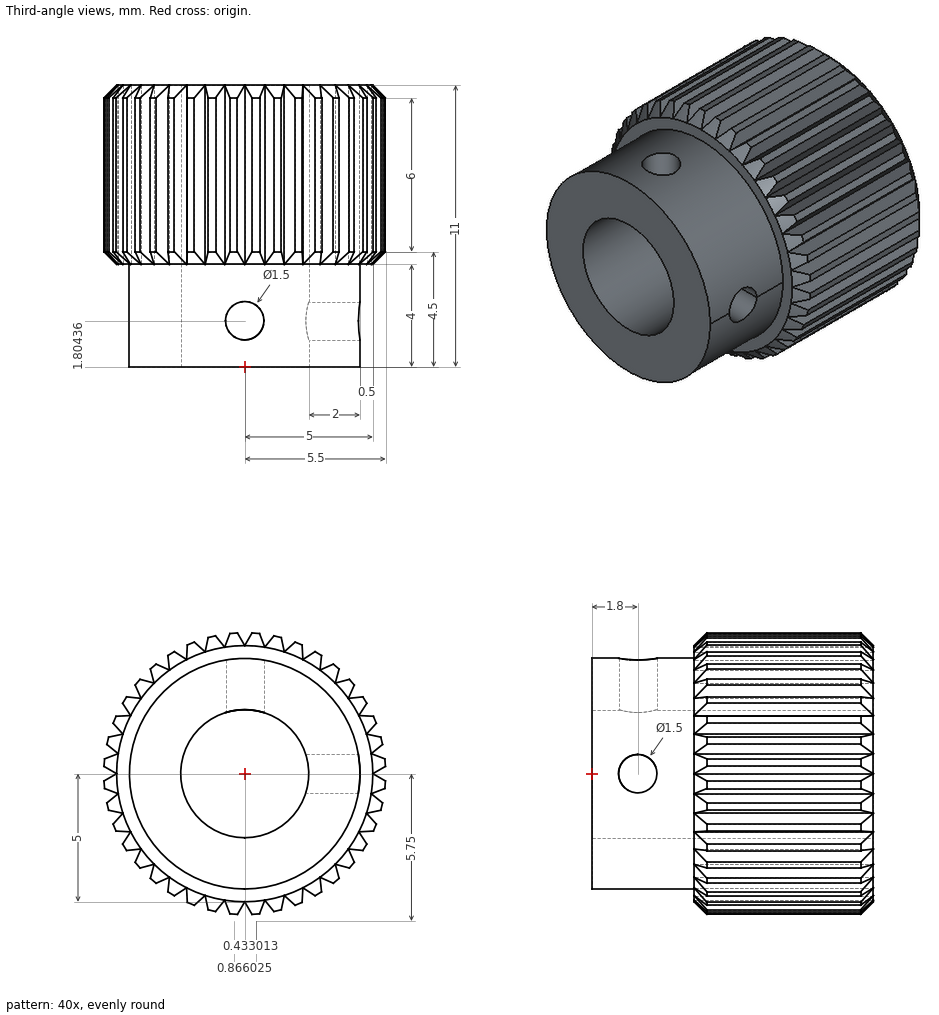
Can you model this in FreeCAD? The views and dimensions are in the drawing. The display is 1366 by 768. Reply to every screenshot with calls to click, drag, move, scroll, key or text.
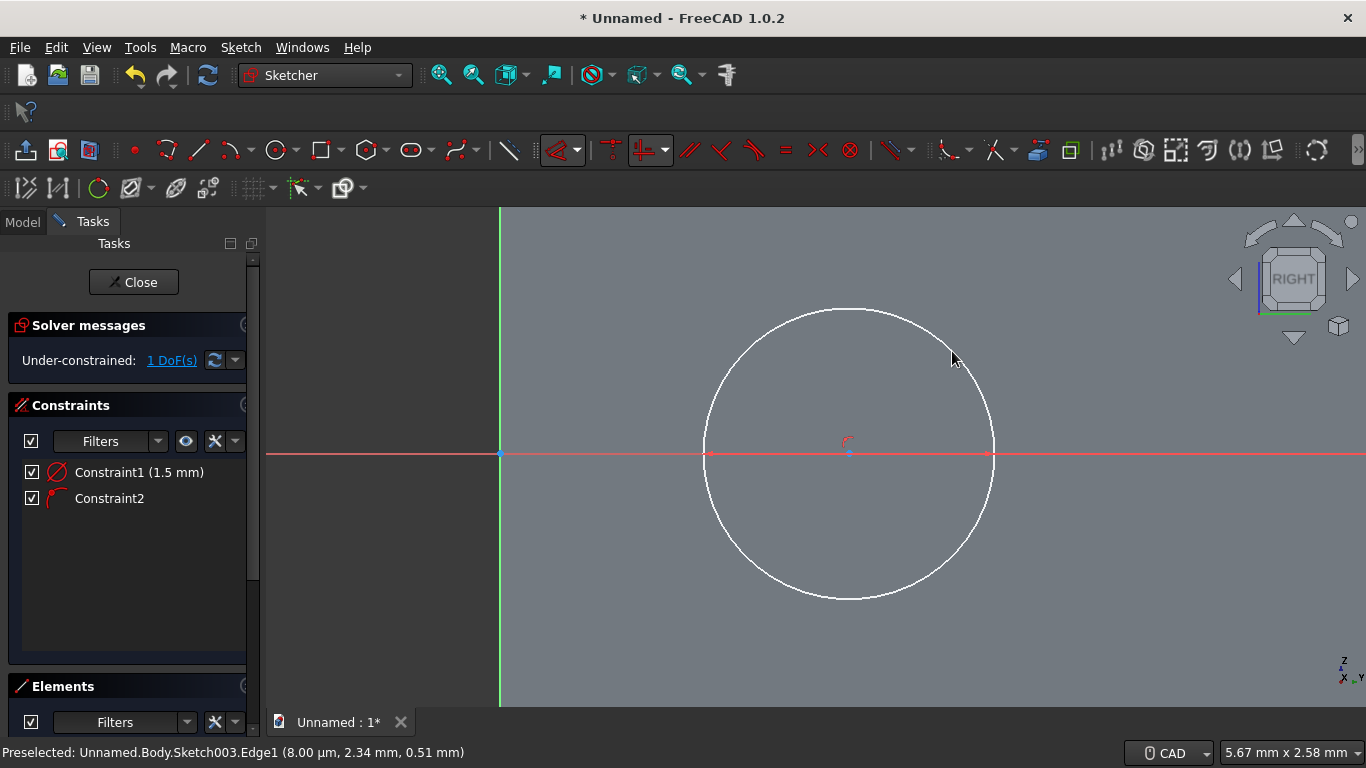
click(849, 454)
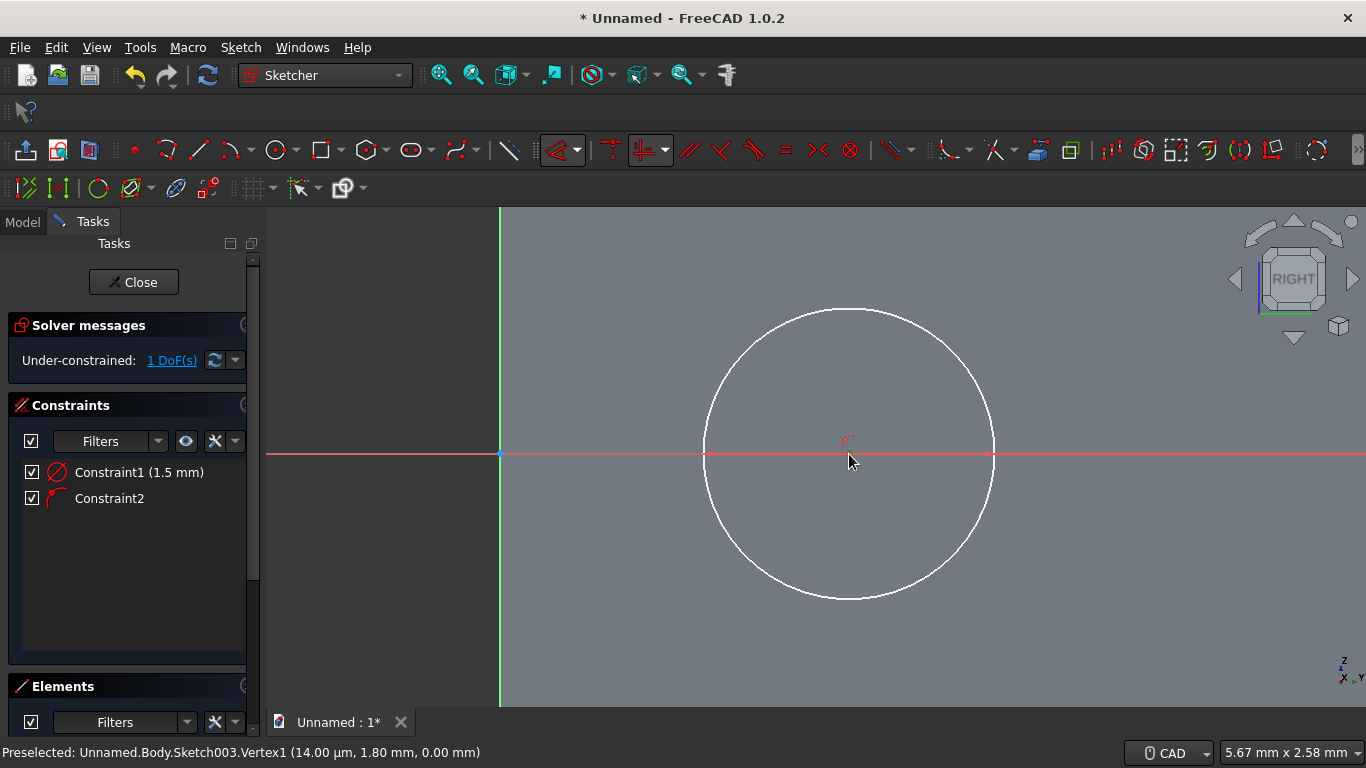
key(l)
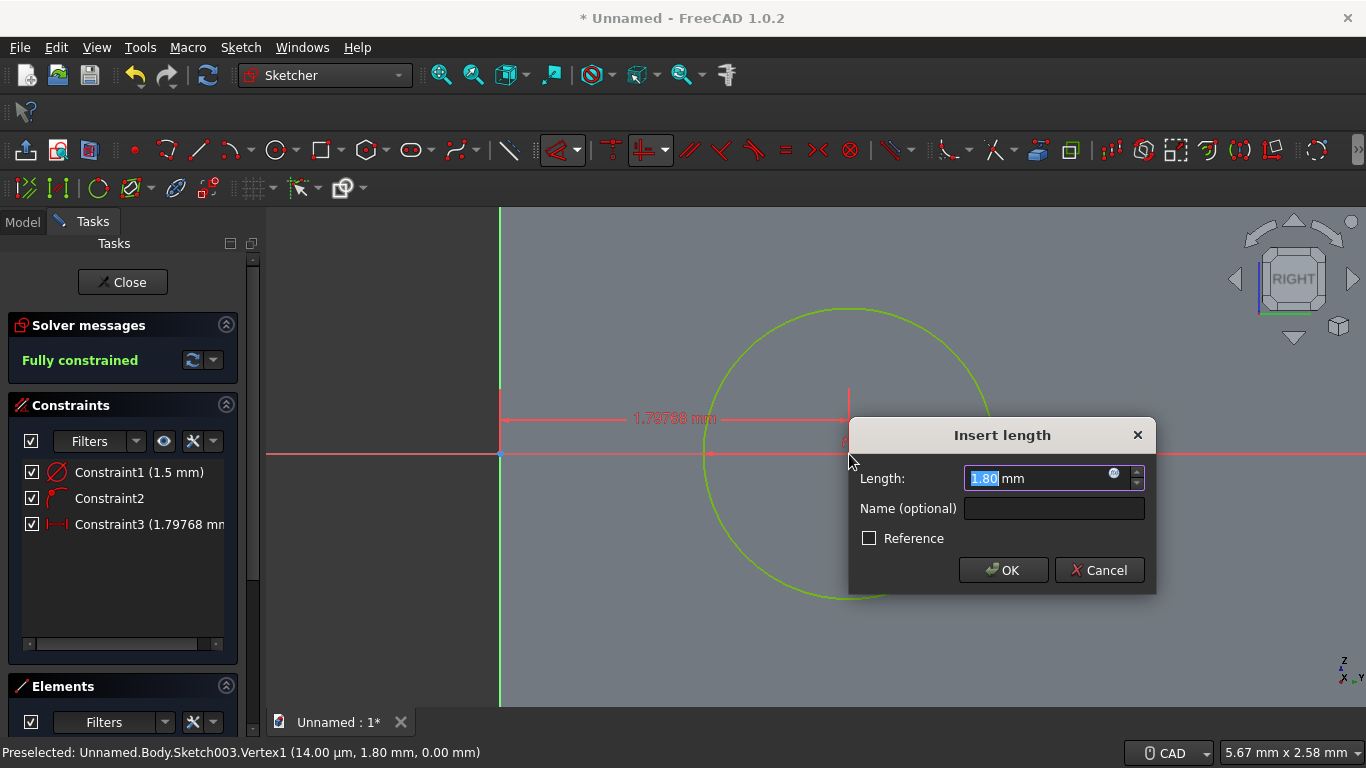
text(1.8)
key(Return)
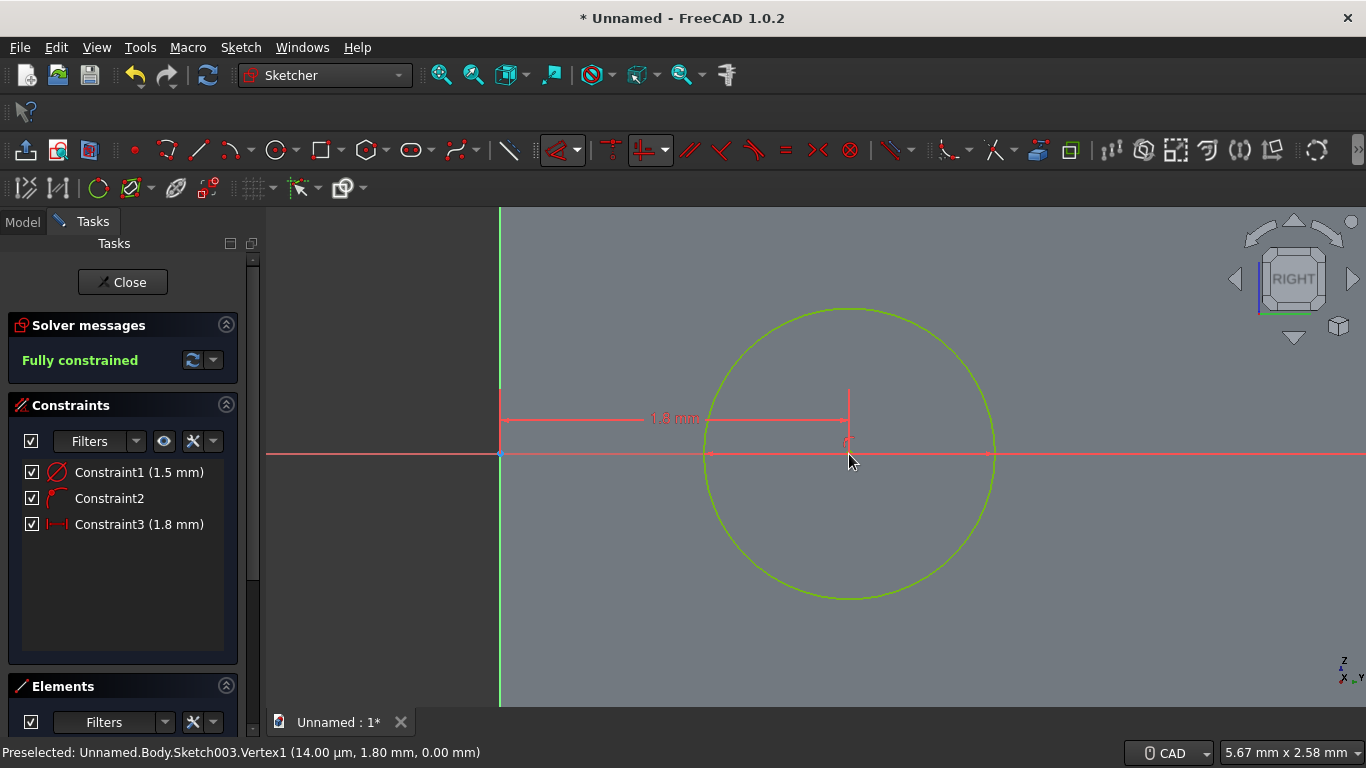
click(123, 282)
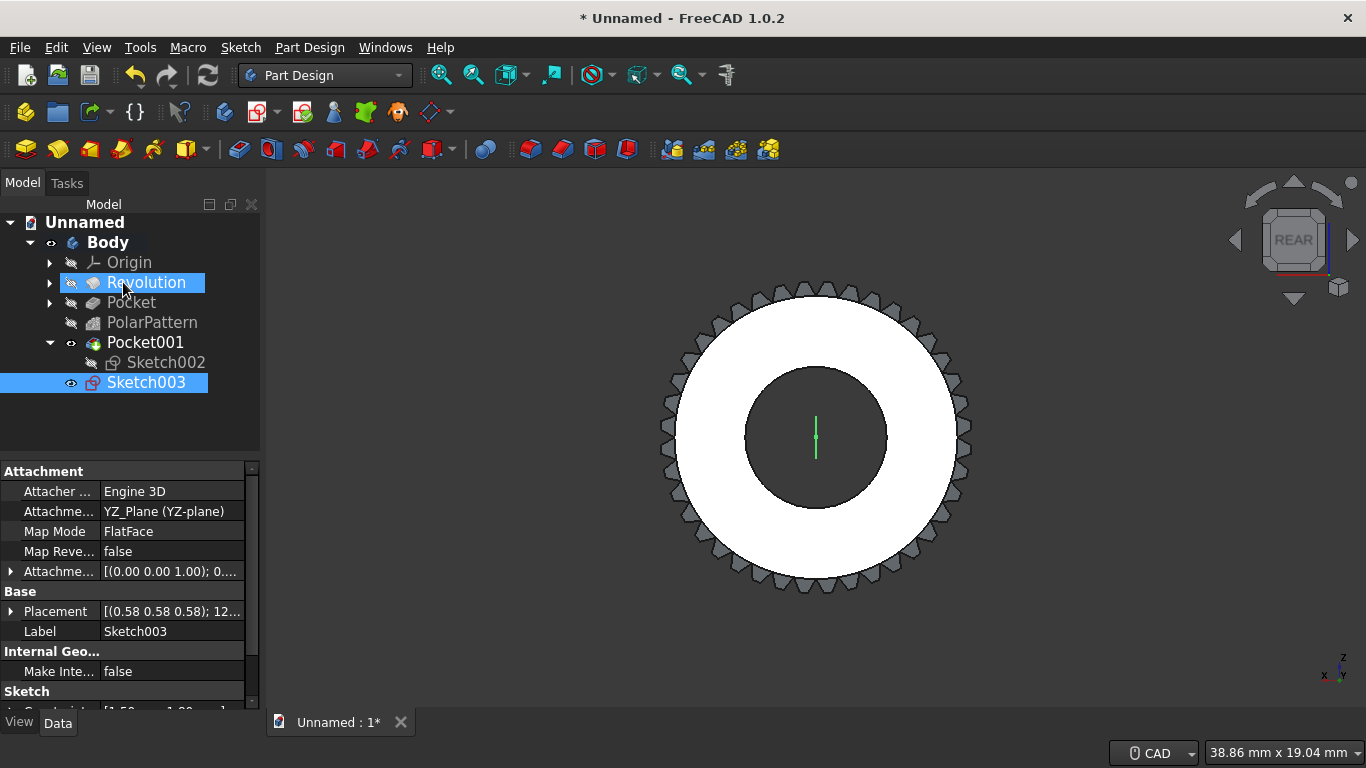
click(240, 150)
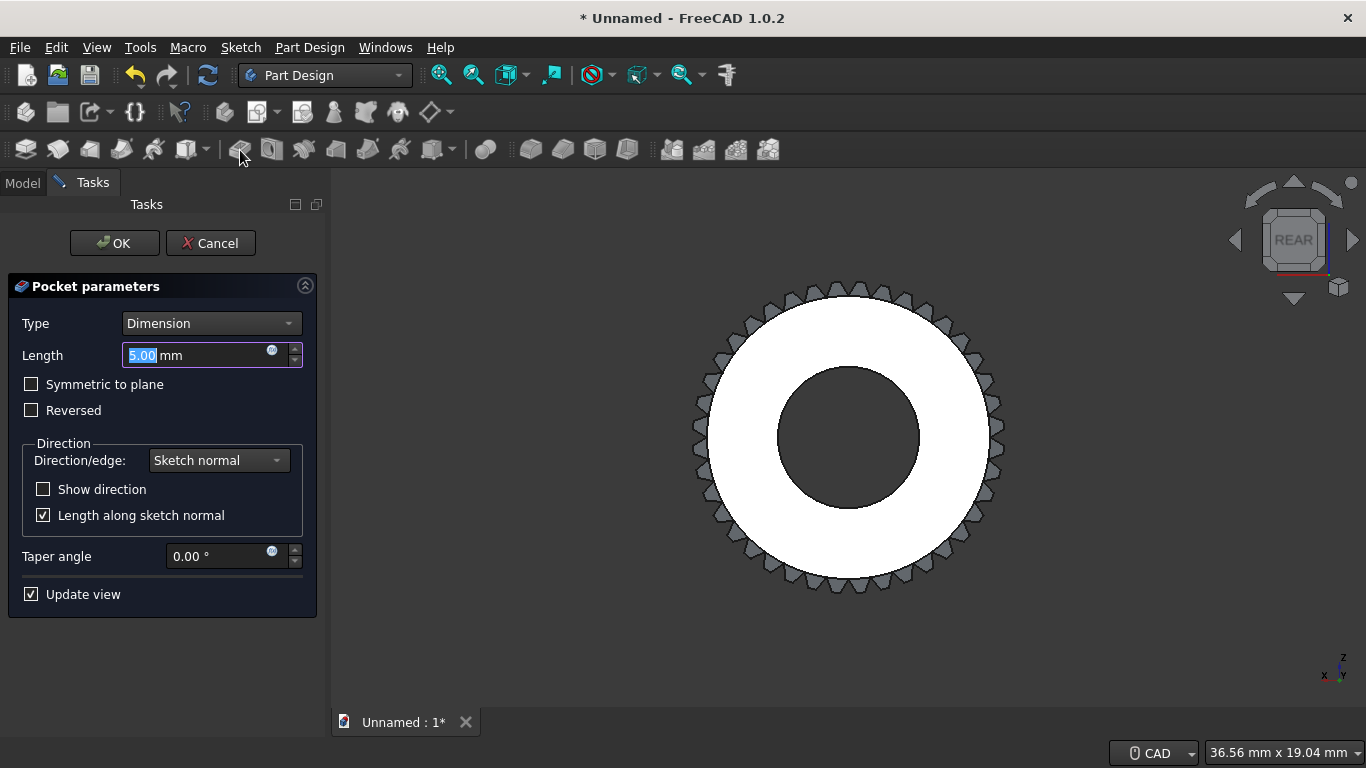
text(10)
key(Tab)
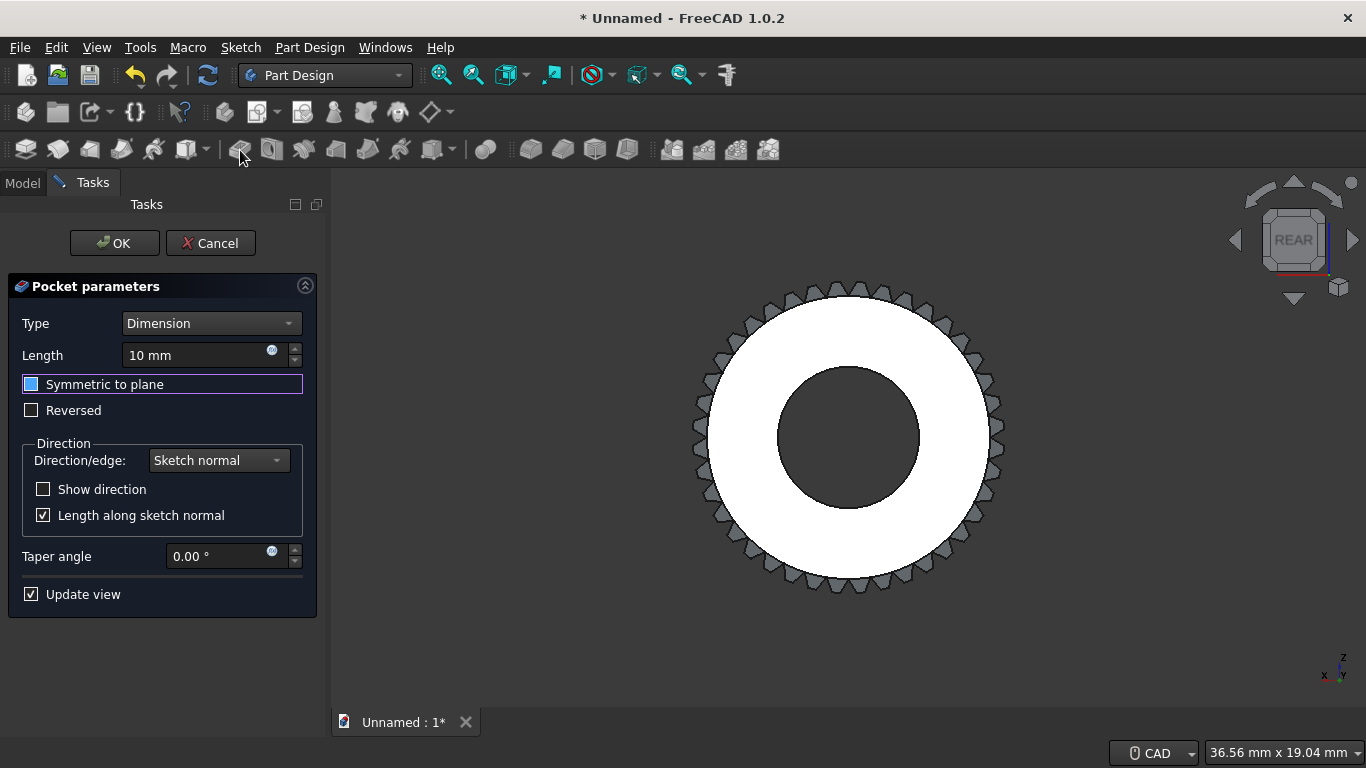
click(30, 410)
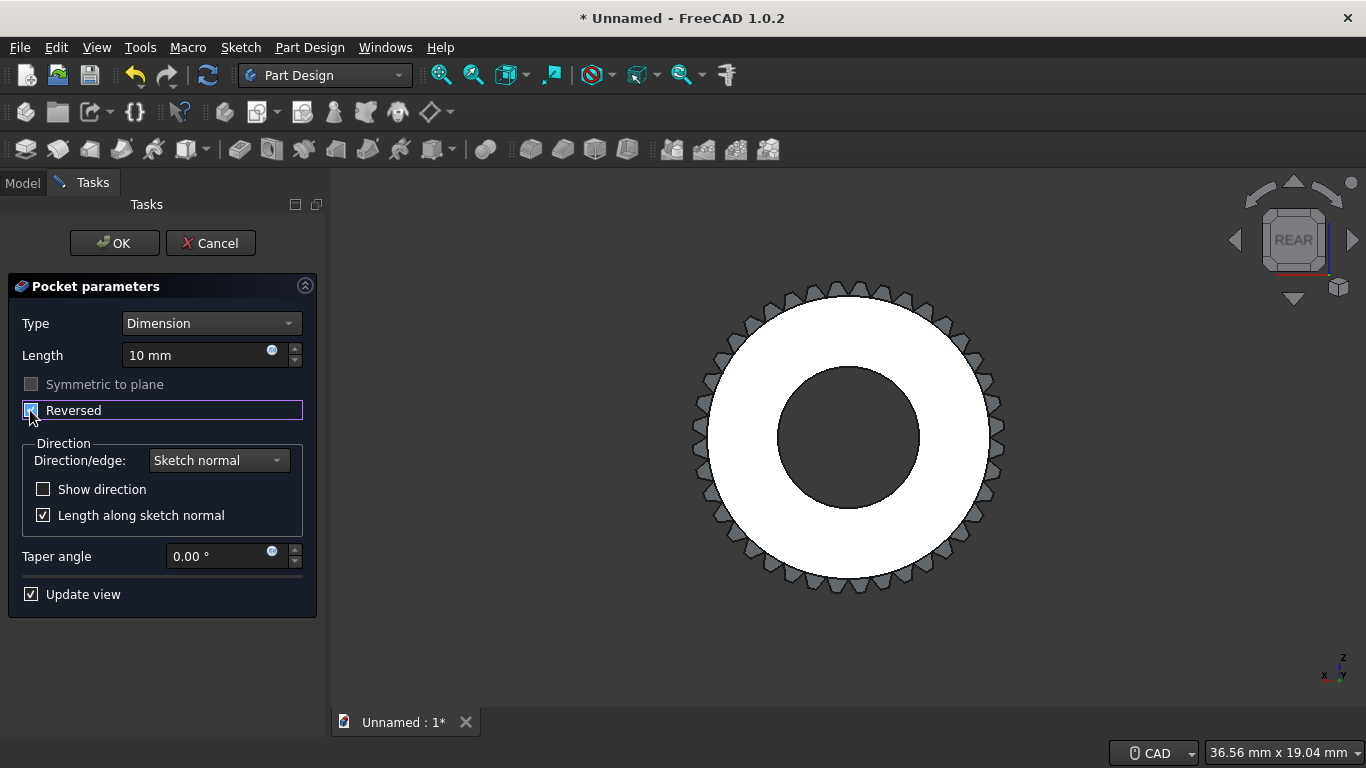
click(115, 243)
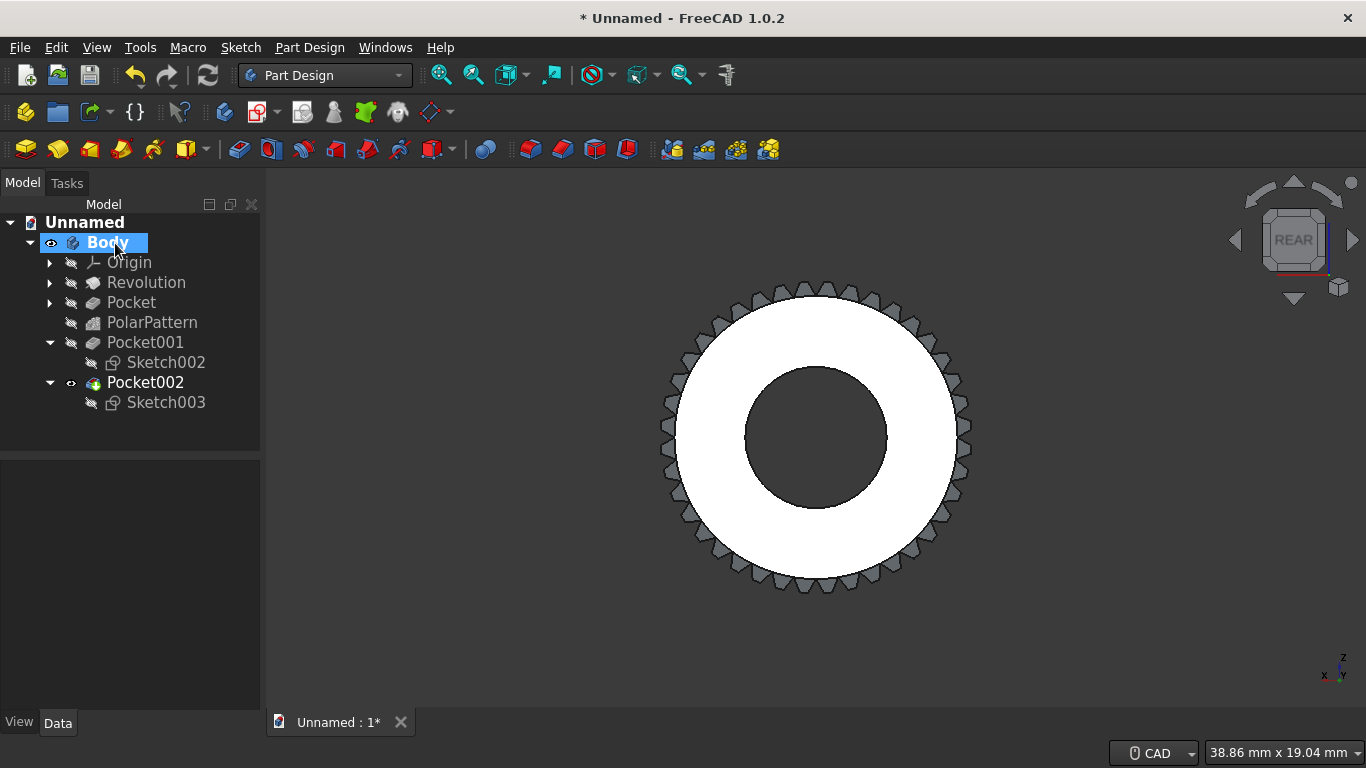
key(0)